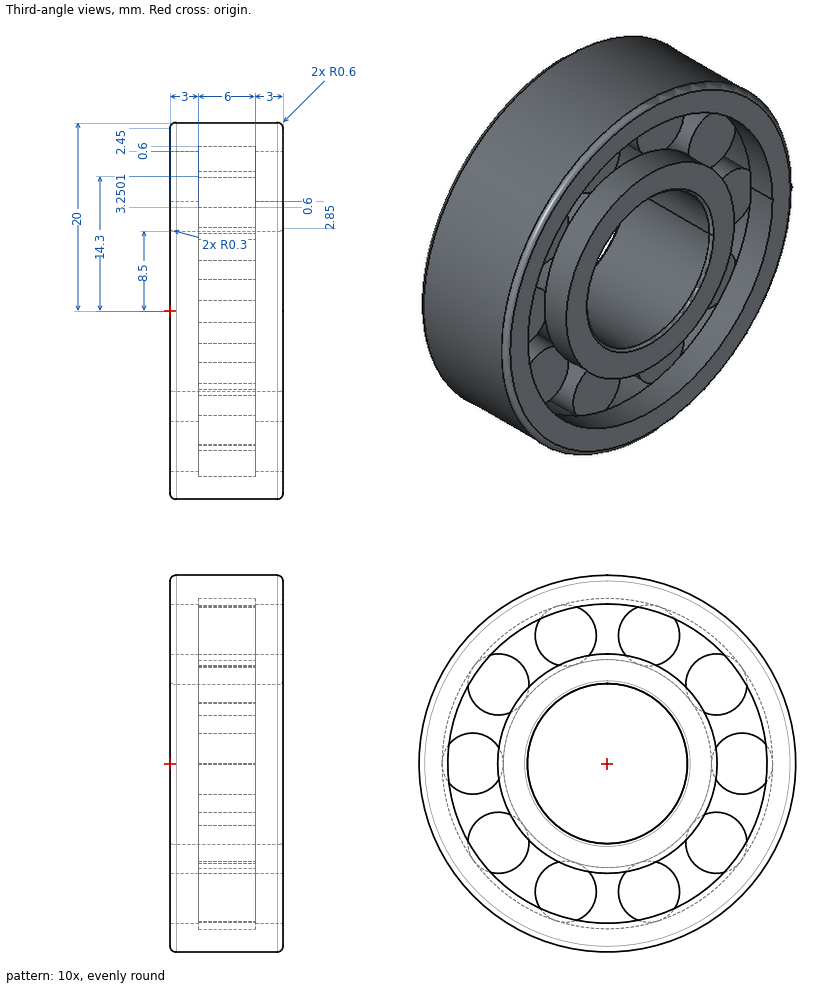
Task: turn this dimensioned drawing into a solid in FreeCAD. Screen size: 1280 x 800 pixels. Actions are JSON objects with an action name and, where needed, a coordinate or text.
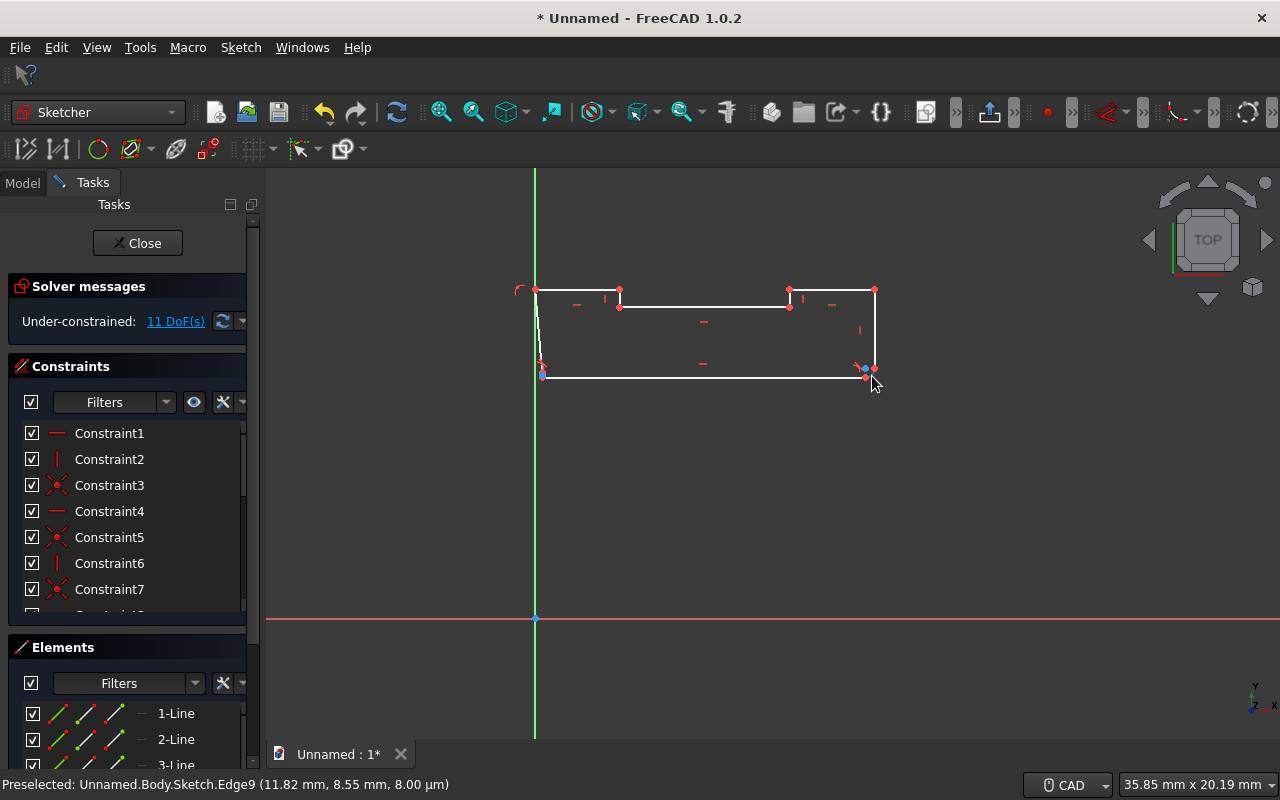
{"action": "scroll", "coordinate": [540, 348], "scroll_direction": "up", "scroll_amount": 6}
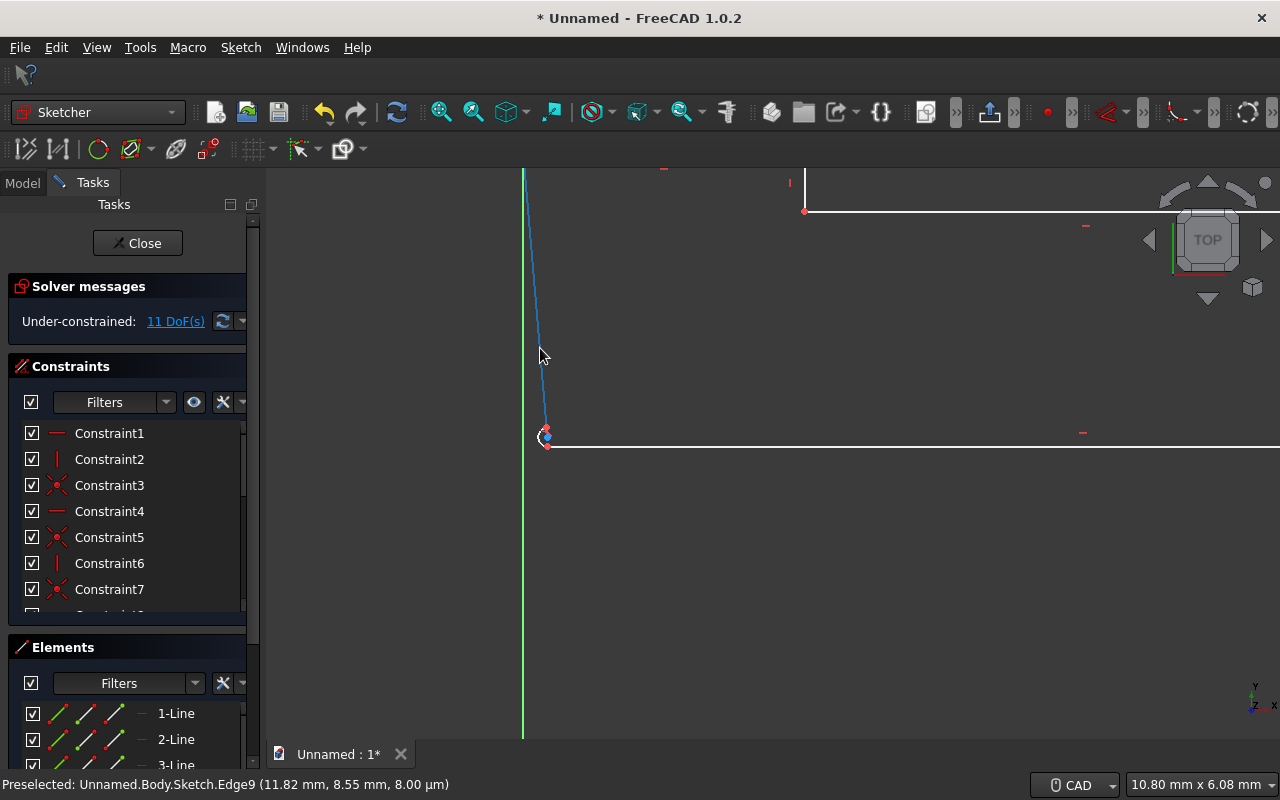
{"action": "left_click", "coordinate": [540, 346]}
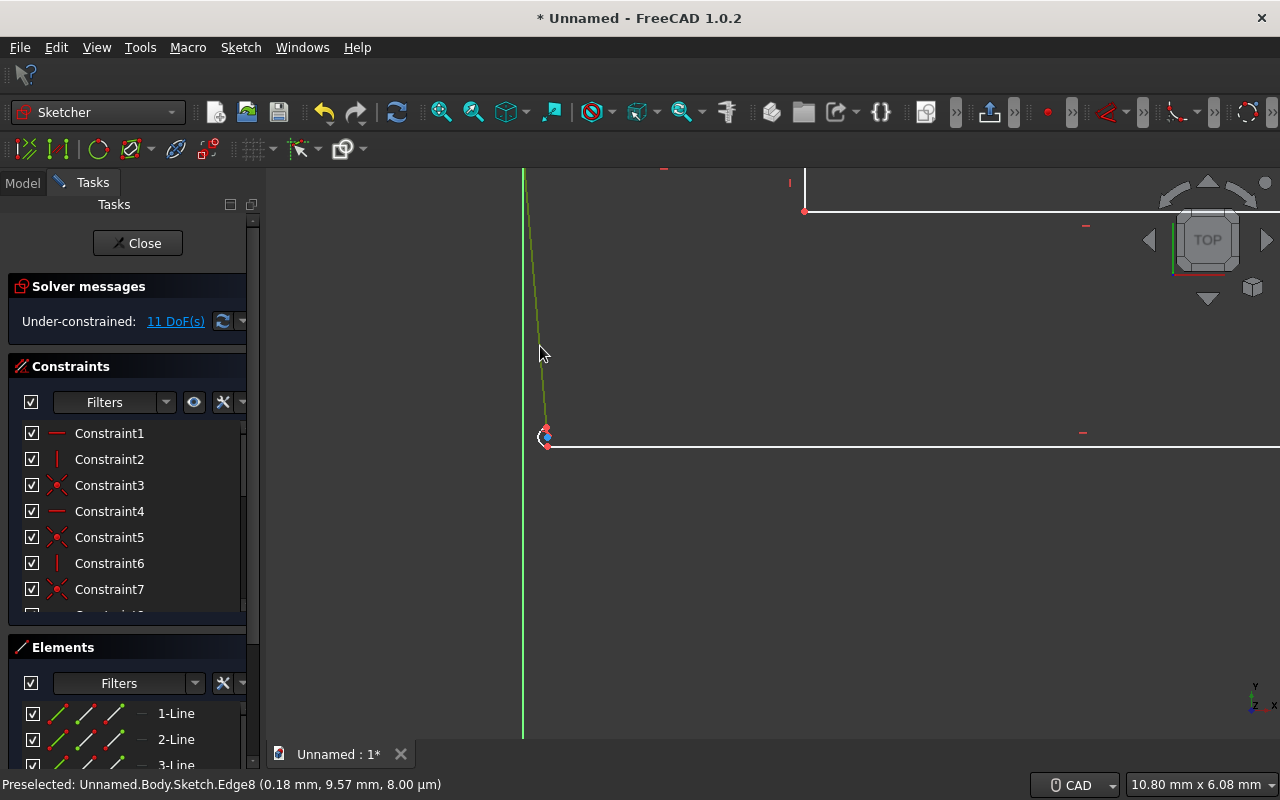
{"action": "scroll", "coordinate": [538, 438], "scroll_direction": "up", "scroll_amount": 2}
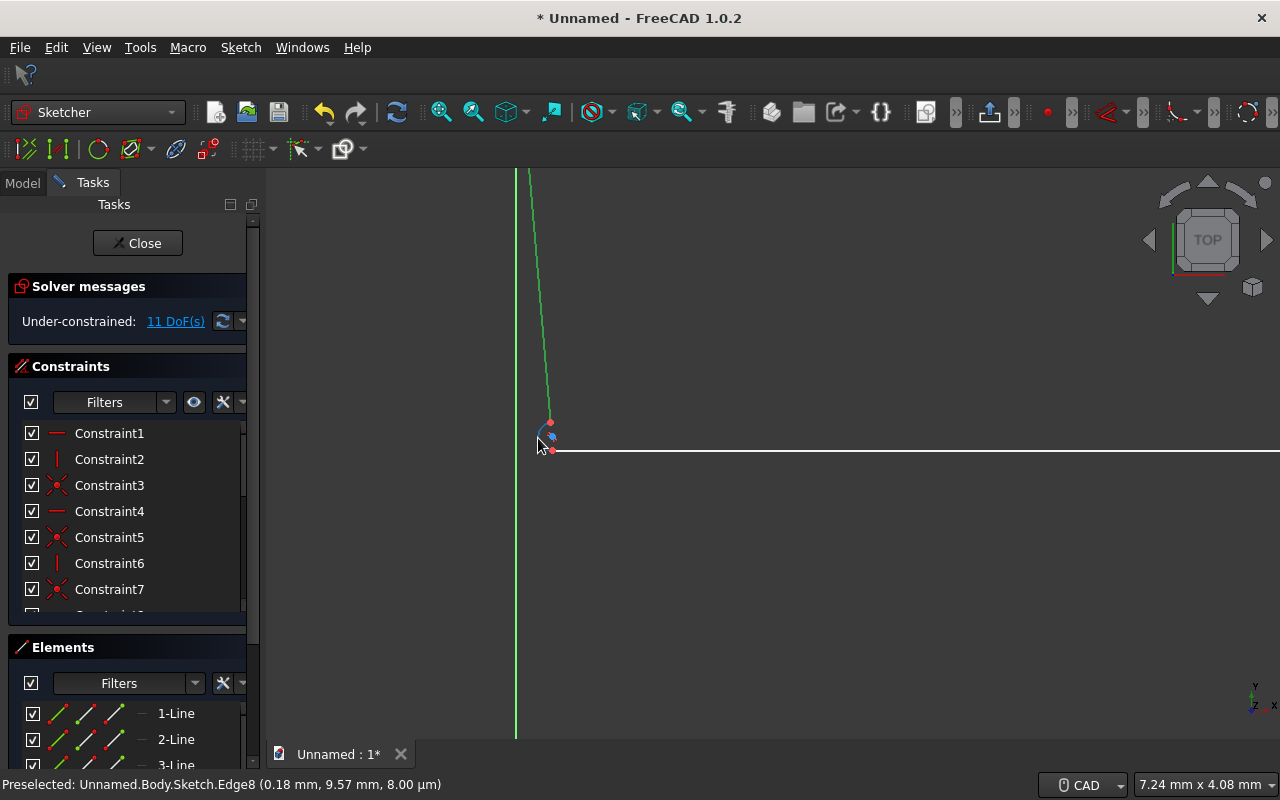
{"action": "left_click", "coordinate": [538, 438]}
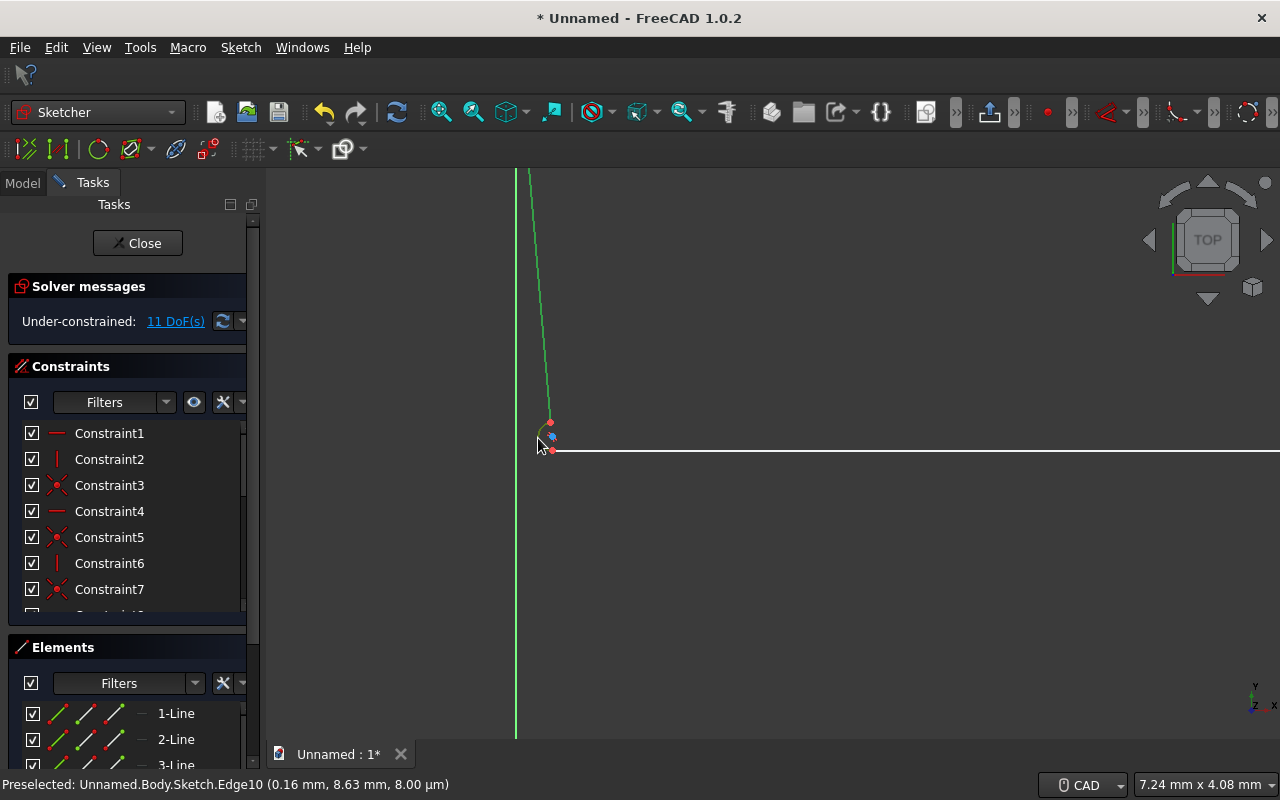
{"action": "key", "text": "t"}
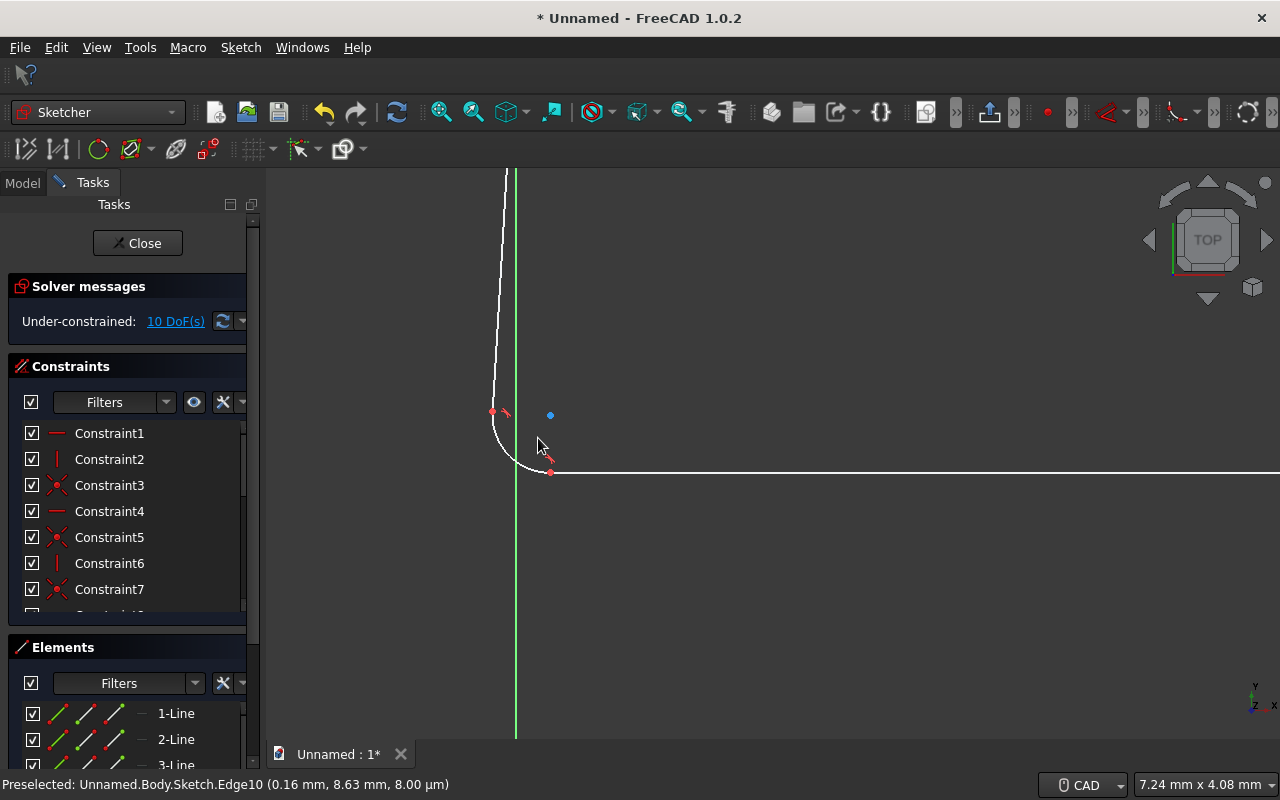
{"action": "left_click", "coordinate": [500, 293]}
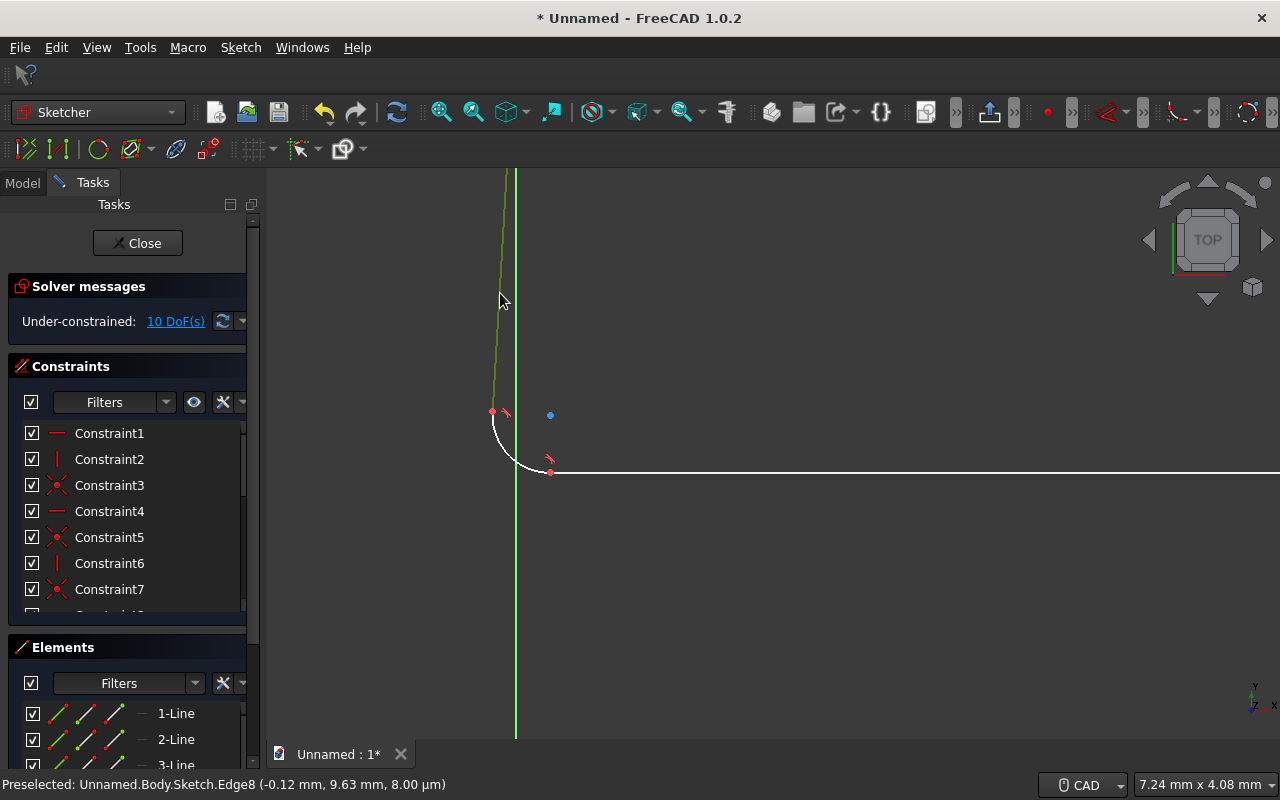
{"action": "key", "text": "v"}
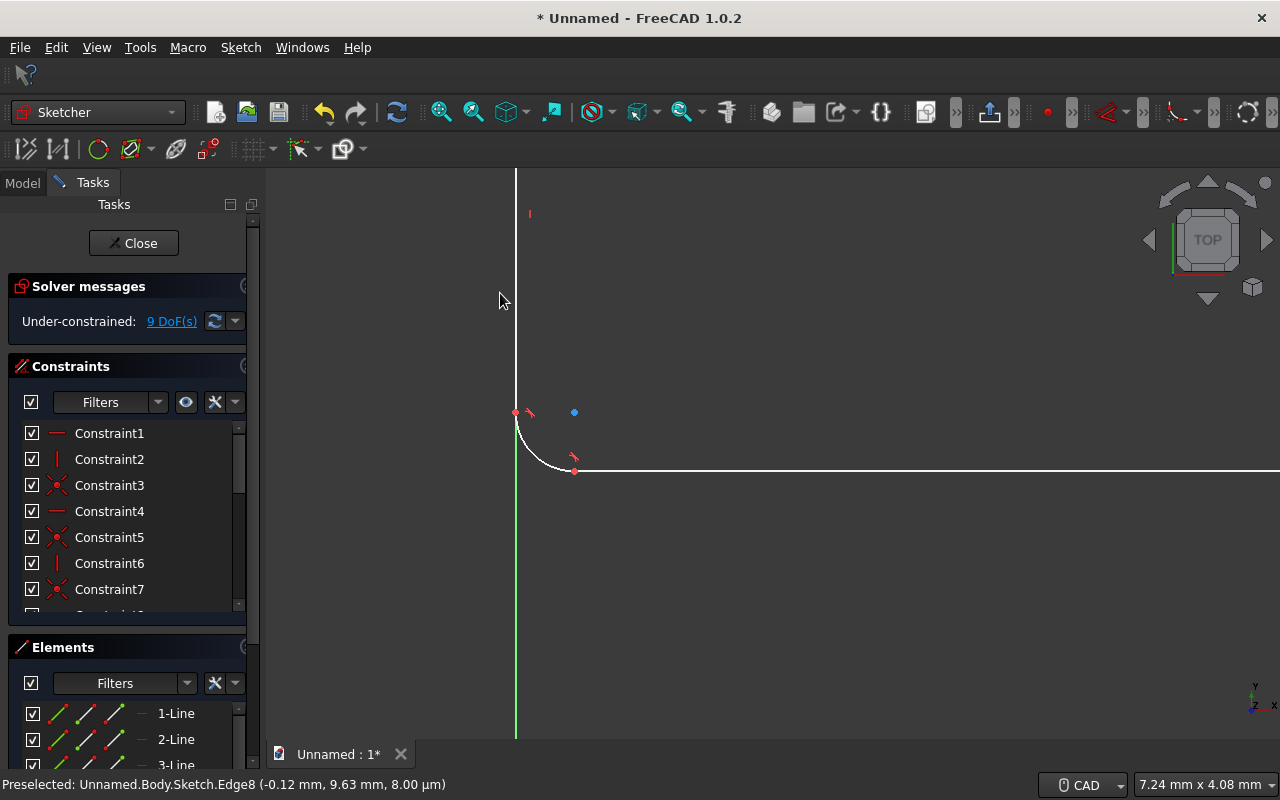
{"action": "scroll", "coordinate": [540, 359], "scroll_direction": "down", "scroll_amount": 8}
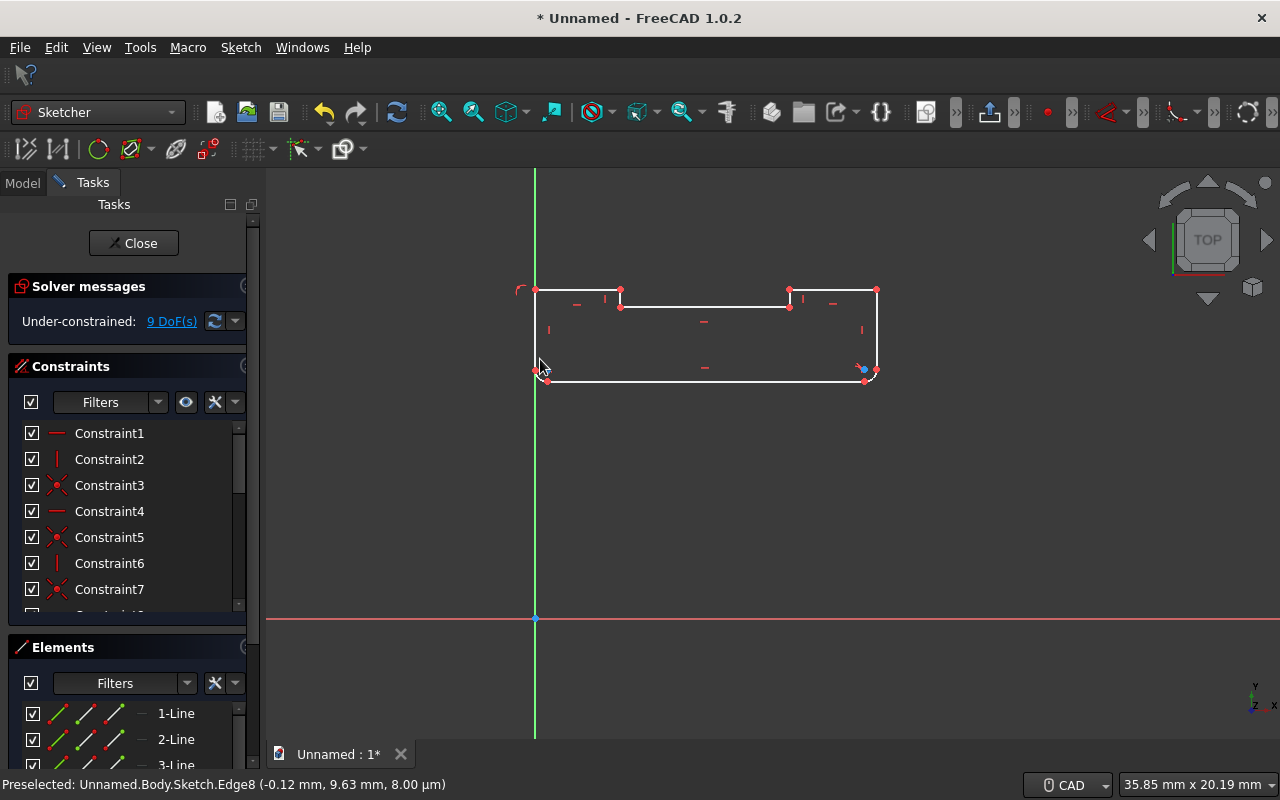
{"action": "scroll", "coordinate": [870, 381], "scroll_direction": "up", "scroll_amount": 5}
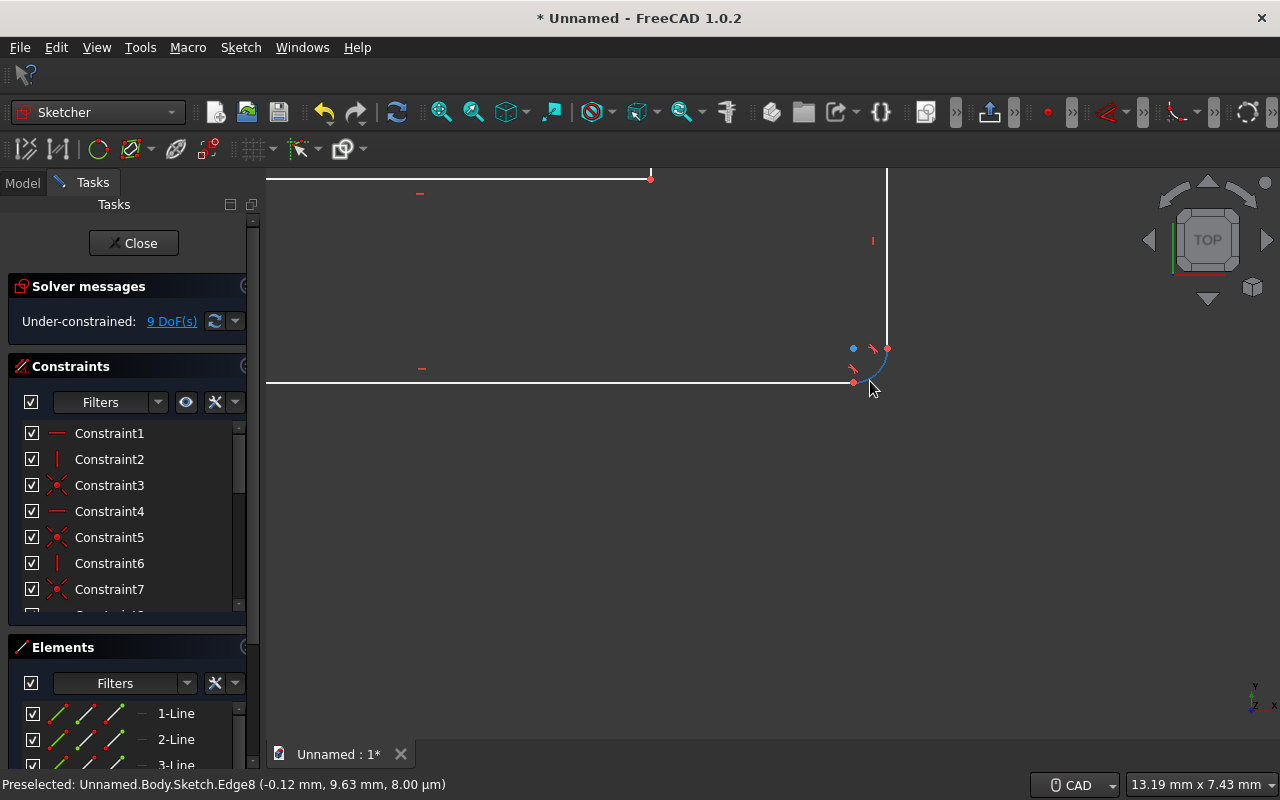
{"action": "left_click", "coordinate": [869, 379]}